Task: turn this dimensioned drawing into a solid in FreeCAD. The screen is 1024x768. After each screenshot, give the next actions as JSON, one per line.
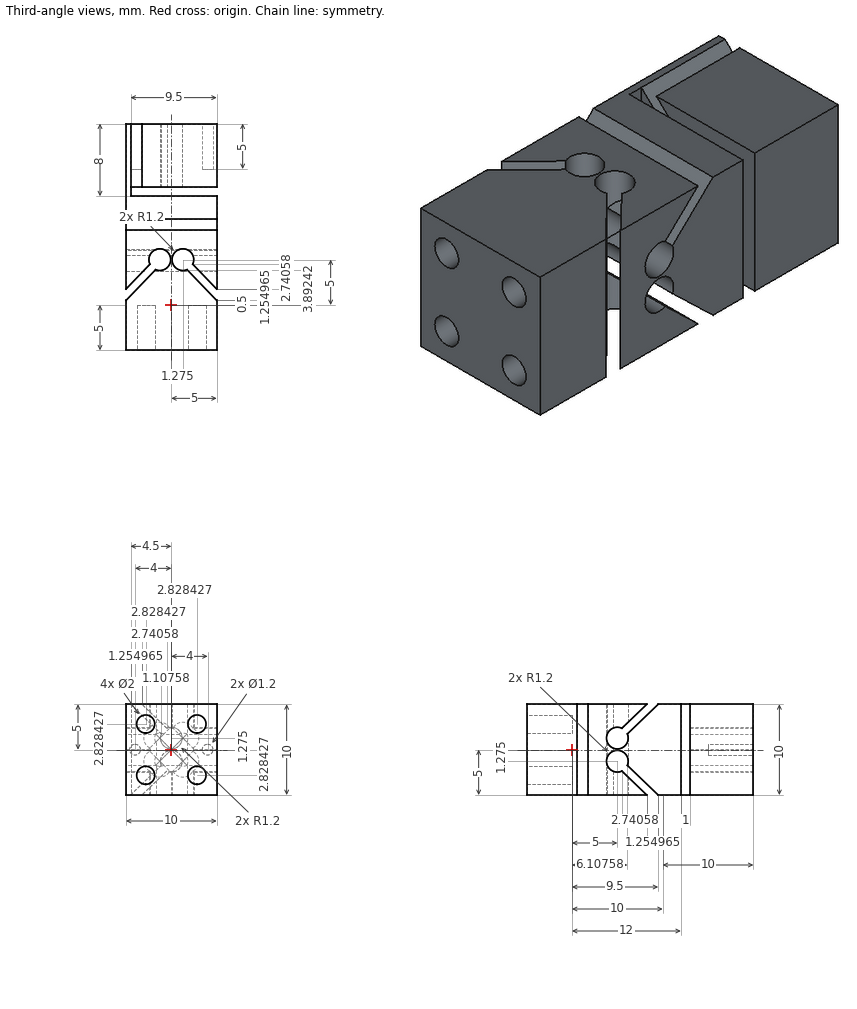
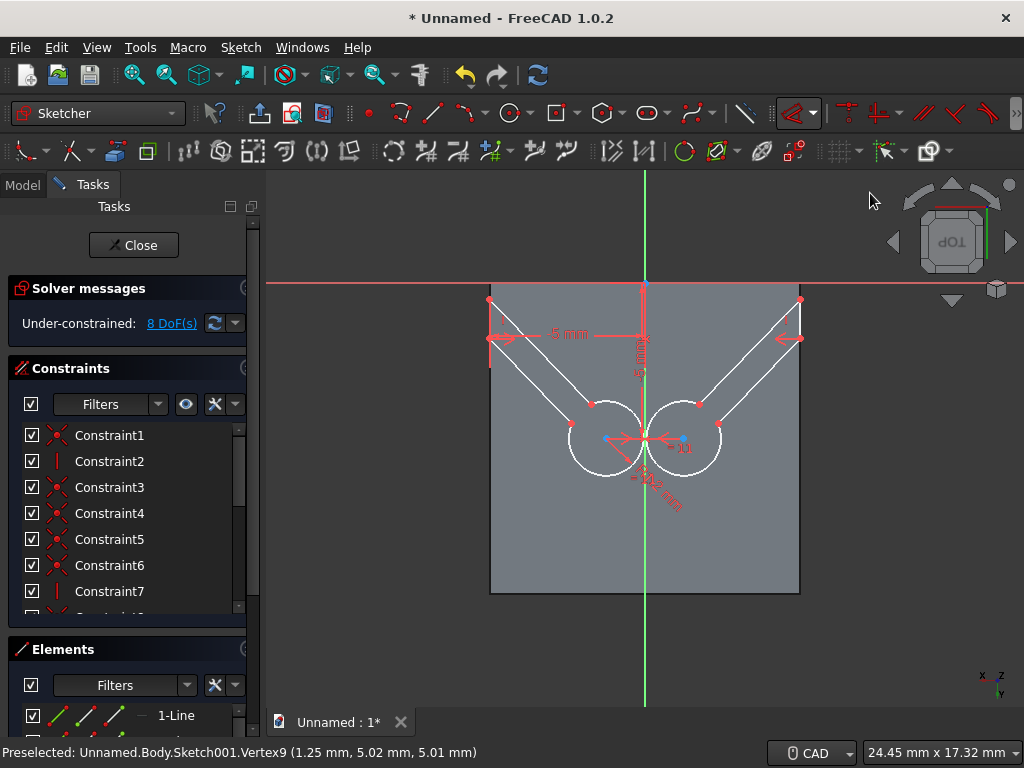
{"action": "scroll", "coordinate": [490, 300], "scroll_direction": "up", "scroll_amount": 5}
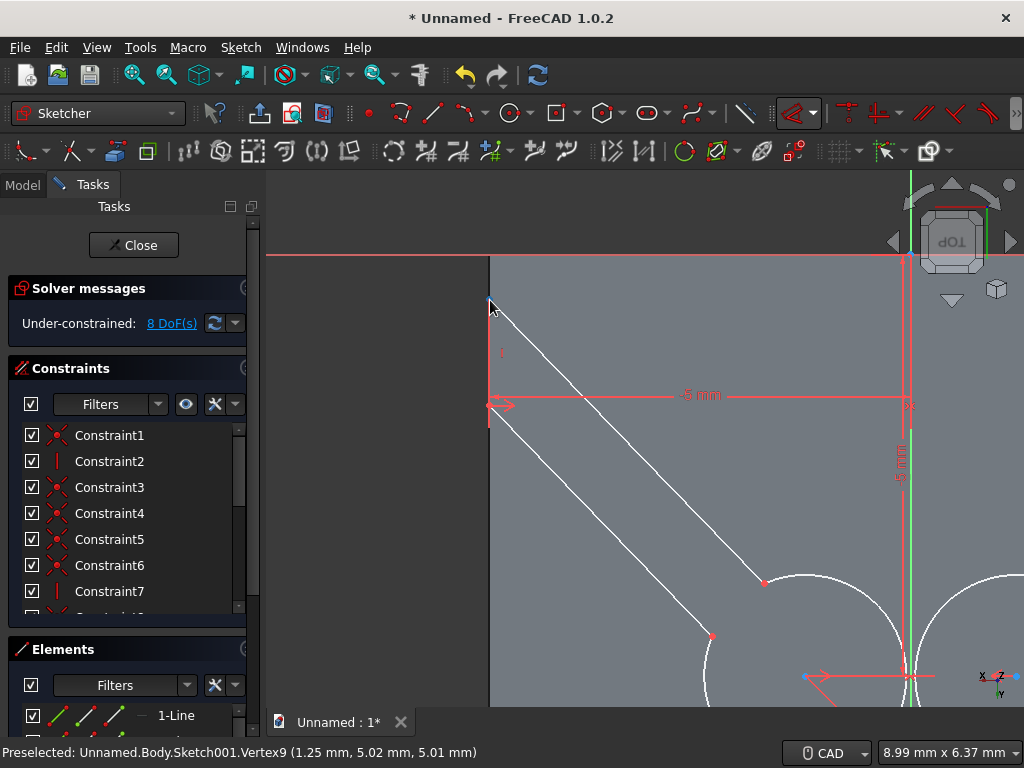
{"action": "left_click", "coordinate": [489, 300]}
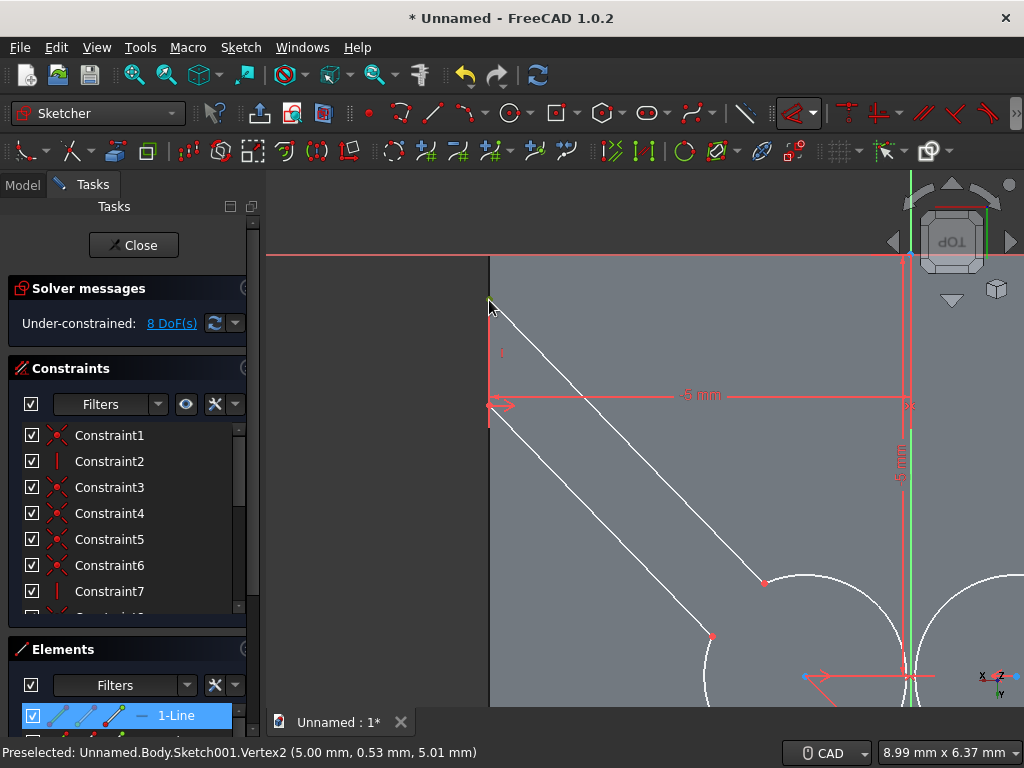
{"action": "left_click", "coordinate": [816, 114]}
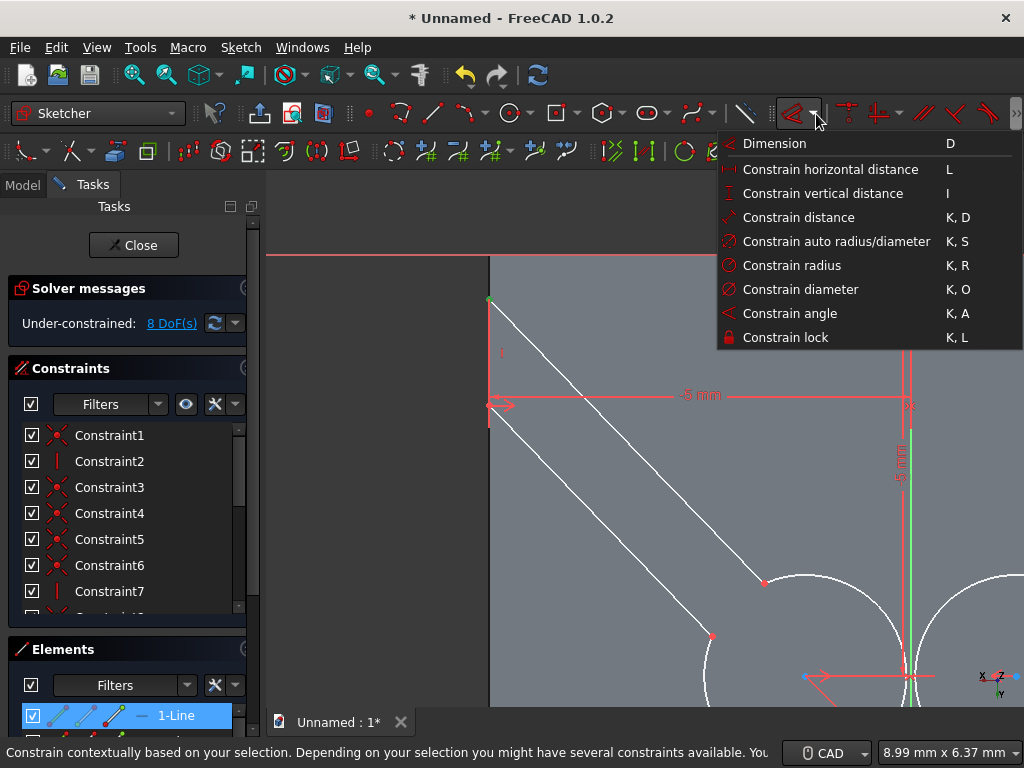
{"action": "left_click", "coordinate": [870, 193]}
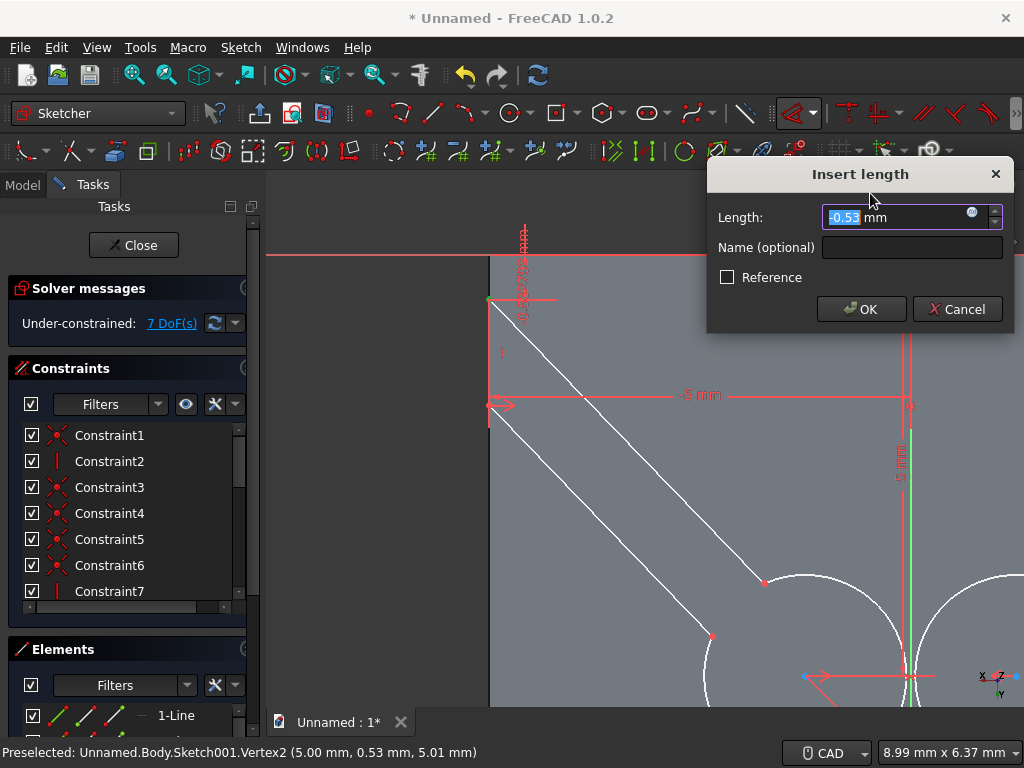
{"action": "type", "text": "-0.5"}
{"action": "key", "text": "Return"}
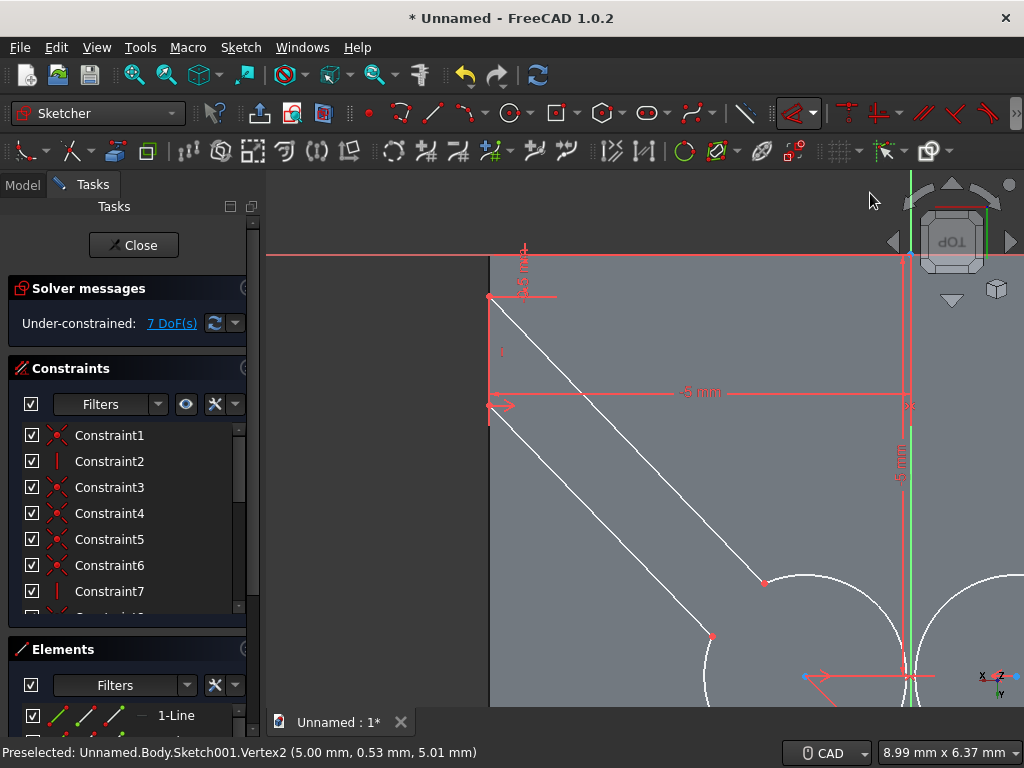
{"action": "scroll", "coordinate": [304, 387], "scroll_direction": "down", "scroll_amount": 4}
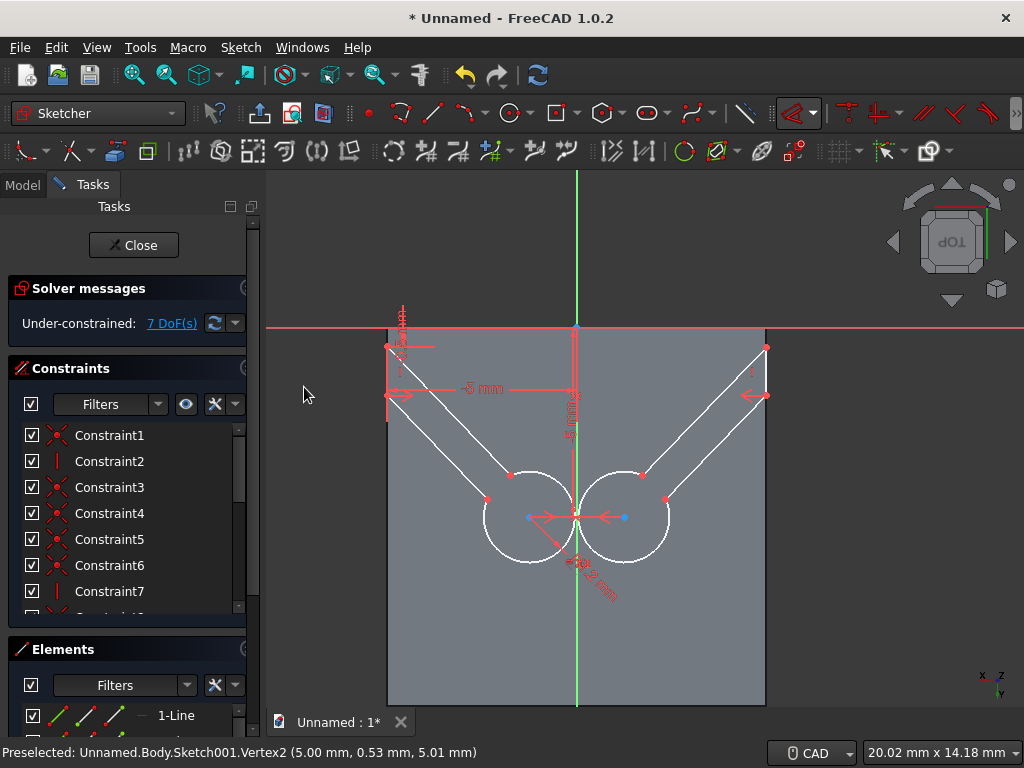
{"action": "scroll", "coordinate": [766, 348], "scroll_direction": "up", "scroll_amount": 4}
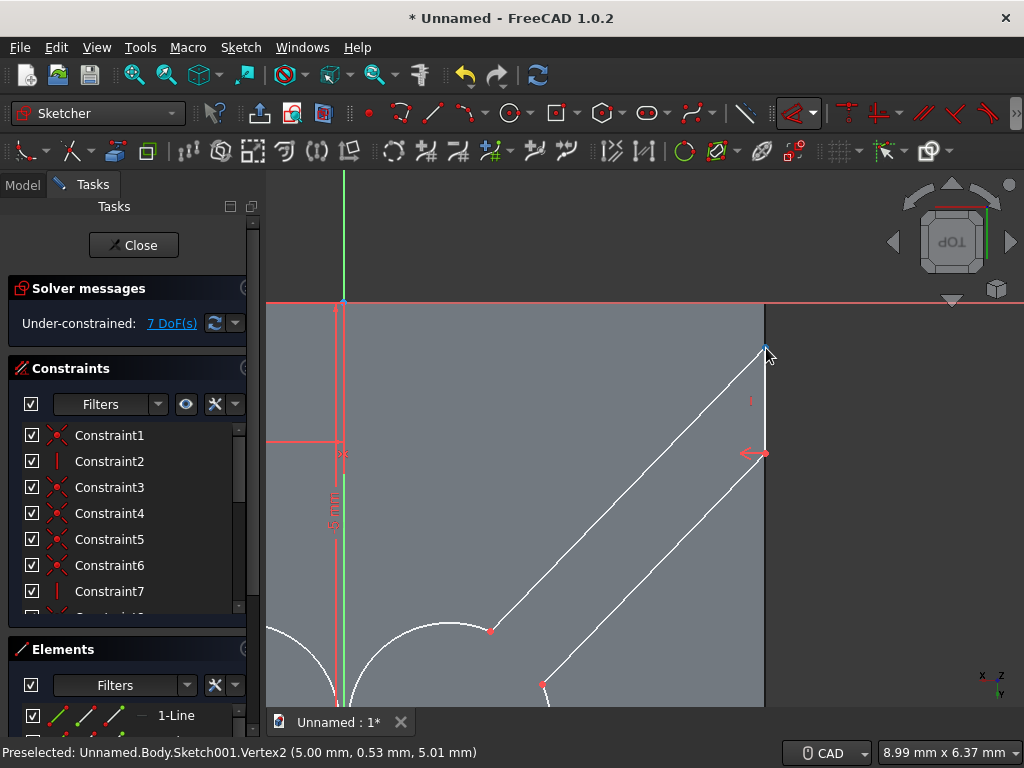
{"action": "left_click", "coordinate": [765, 347]}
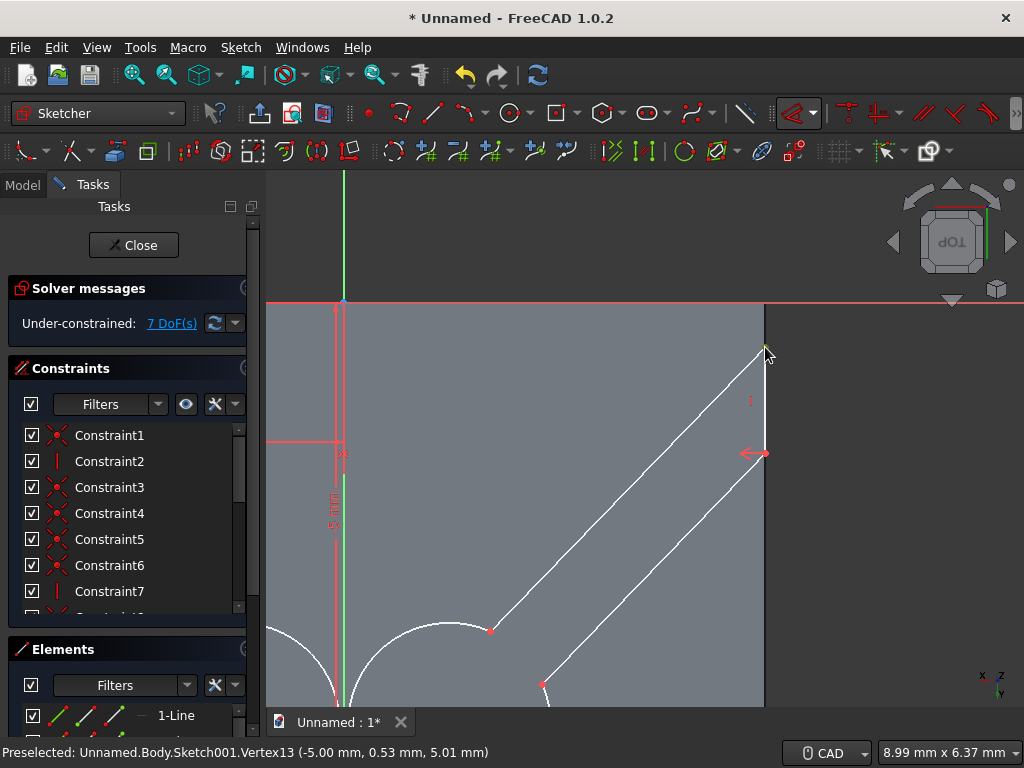
{"action": "left_click", "coordinate": [816, 114]}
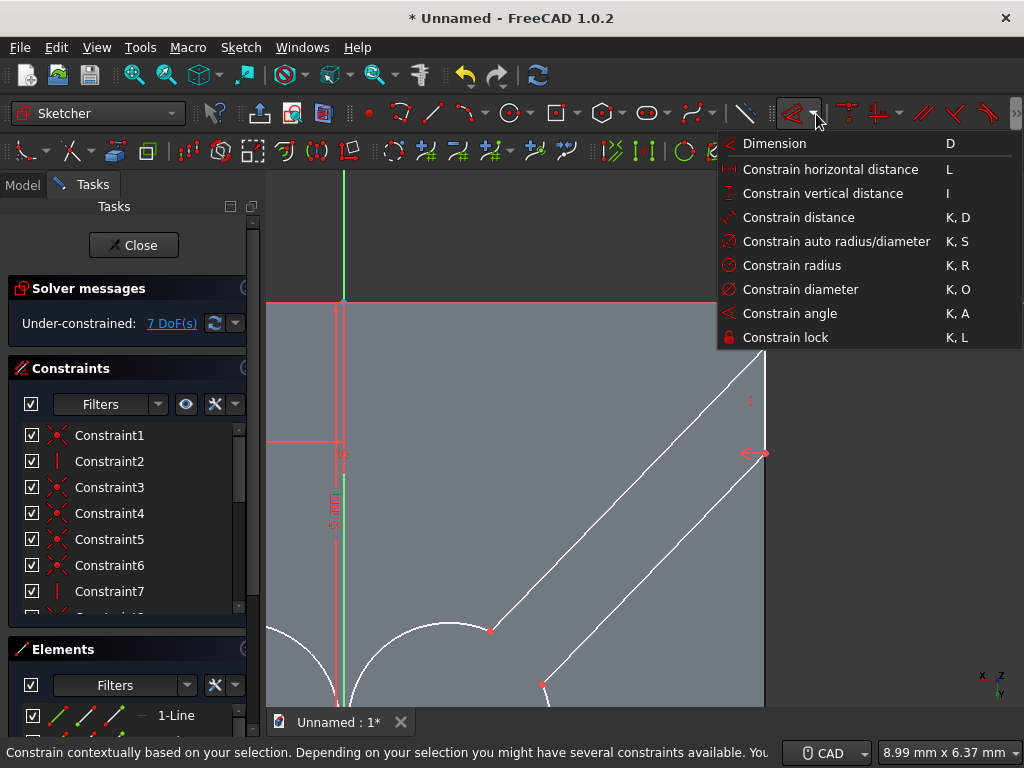
{"action": "left_click", "coordinate": [870, 193]}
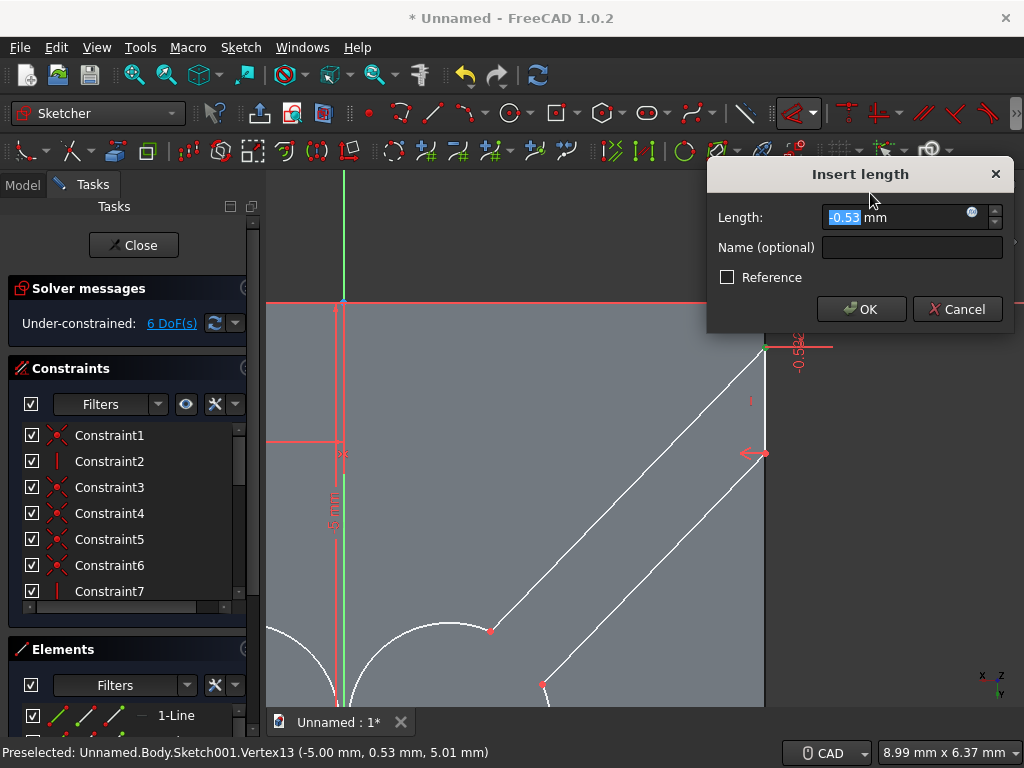
{"action": "type", "text": "-0.5"}
{"action": "key", "text": "Return"}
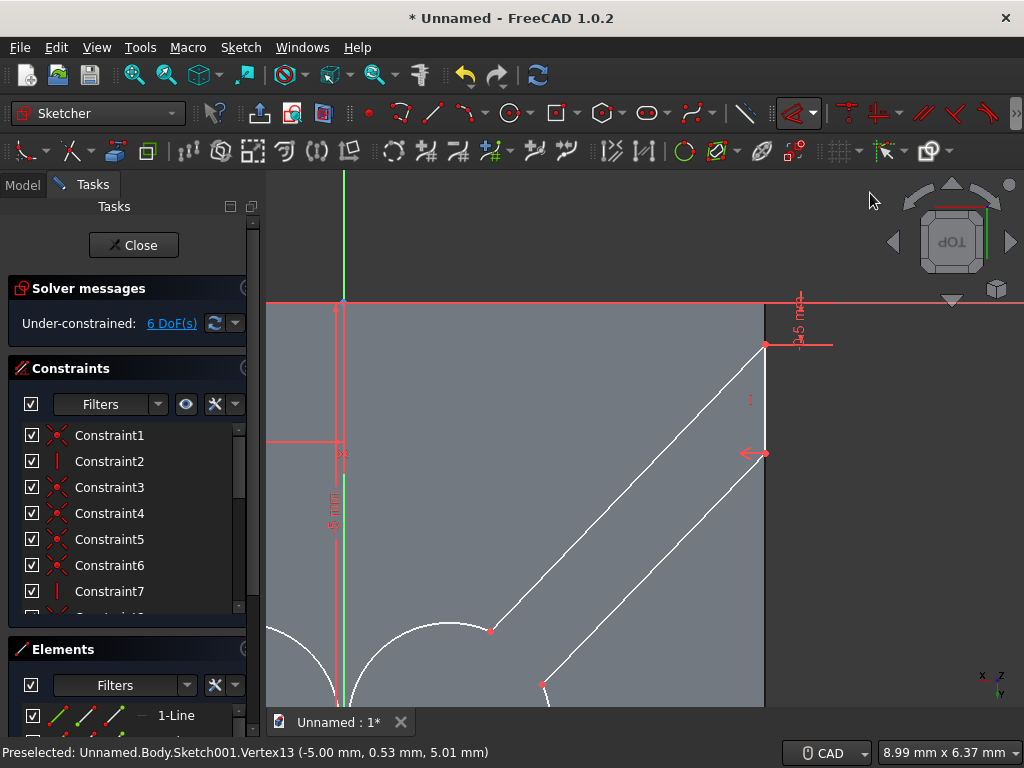
{"action": "scroll", "coordinate": [766, 348], "scroll_direction": "down", "scroll_amount": 4}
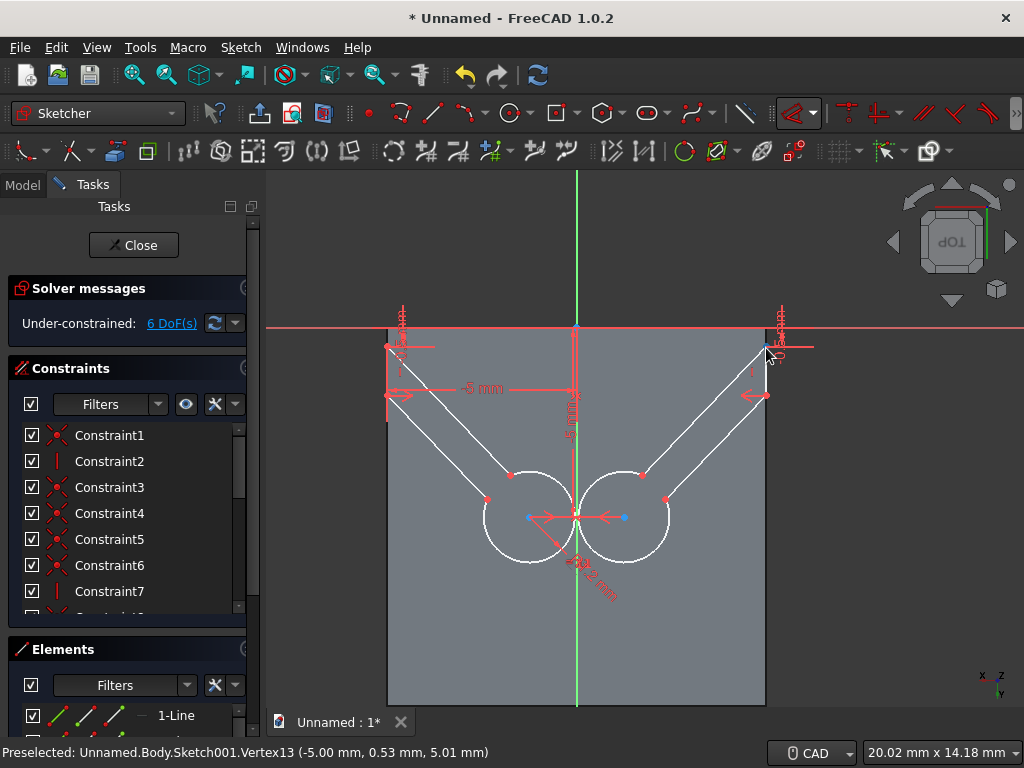
{"action": "left_click", "coordinate": [529, 517]}